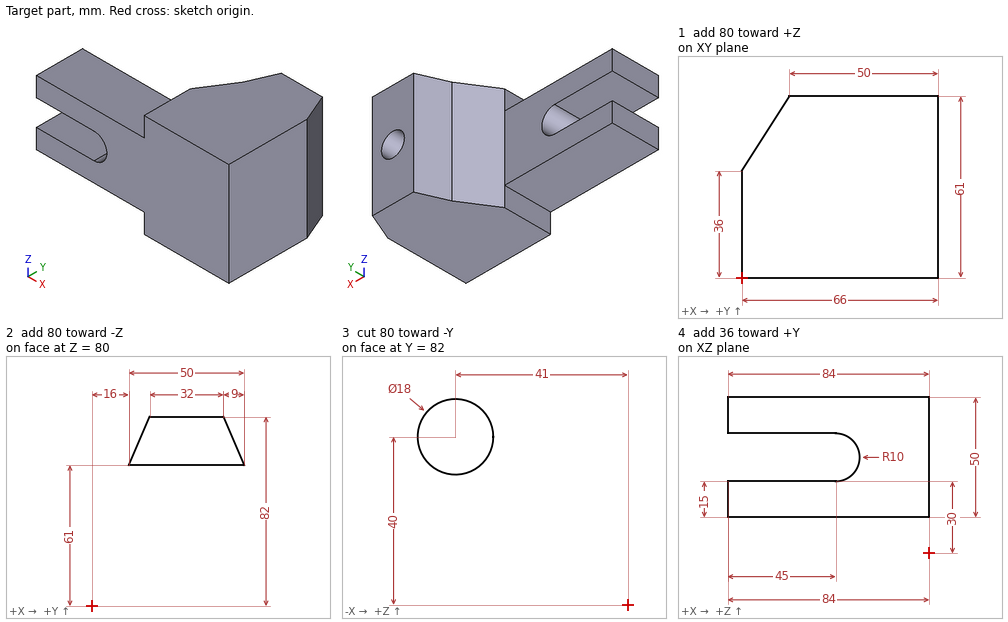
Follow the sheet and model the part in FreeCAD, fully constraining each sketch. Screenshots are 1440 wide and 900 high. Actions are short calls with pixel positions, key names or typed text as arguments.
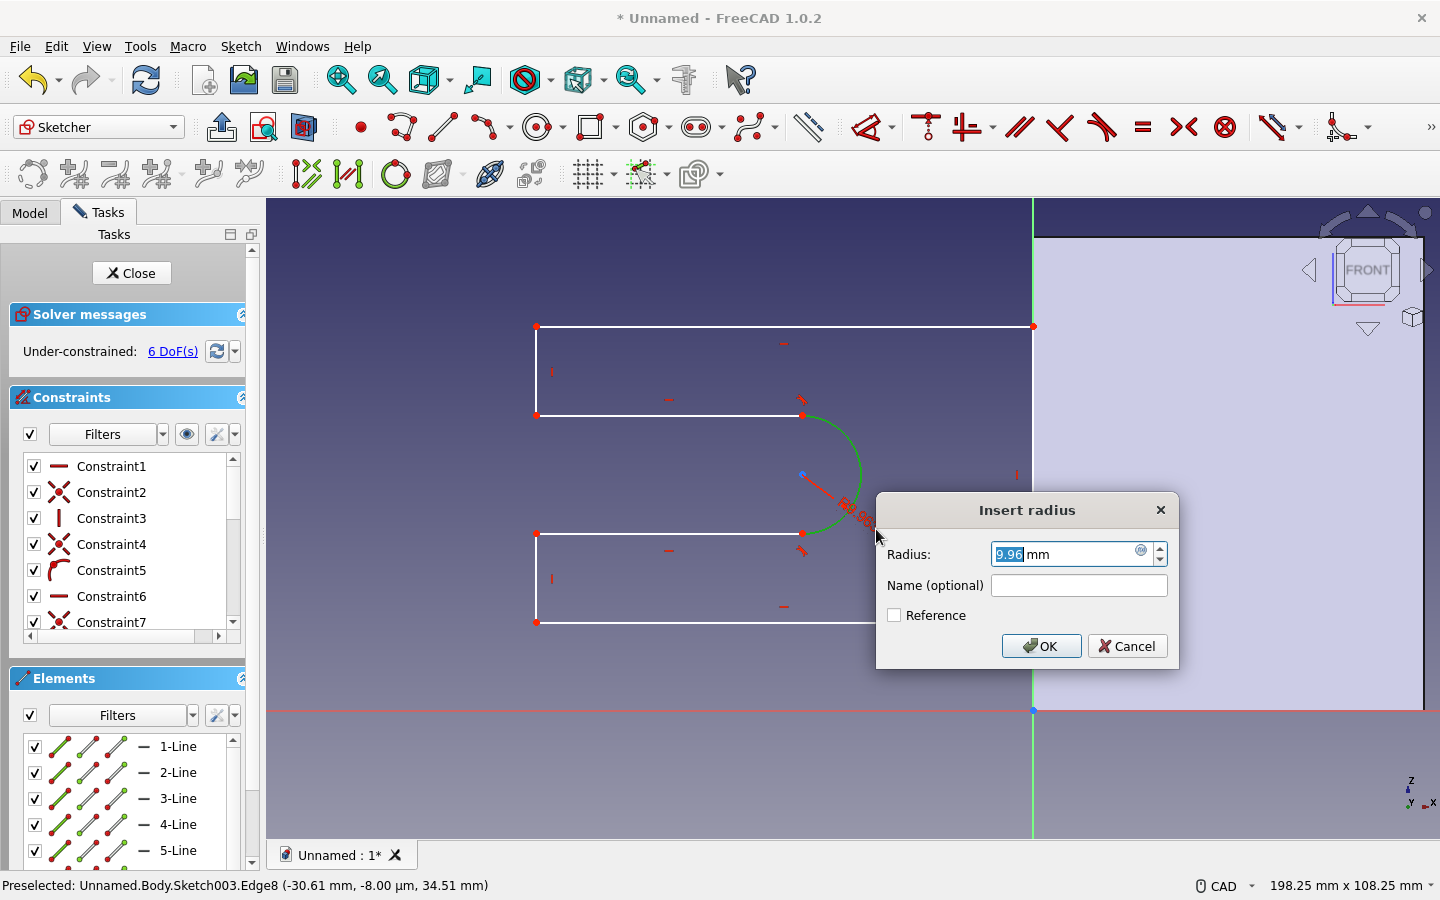
text(10)
key(Return)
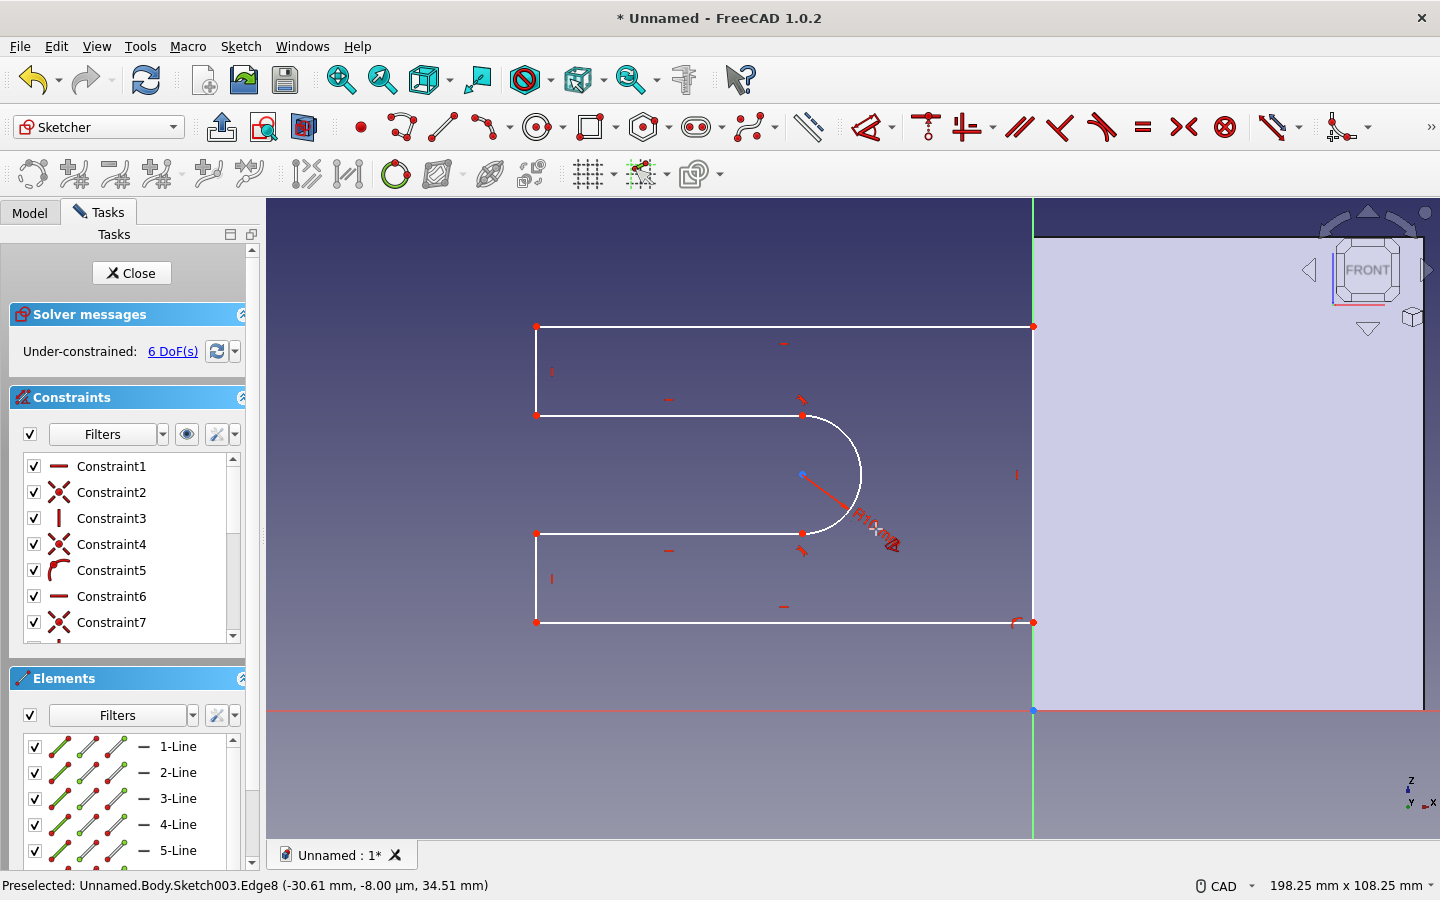
click(722, 534)
click(669, 568)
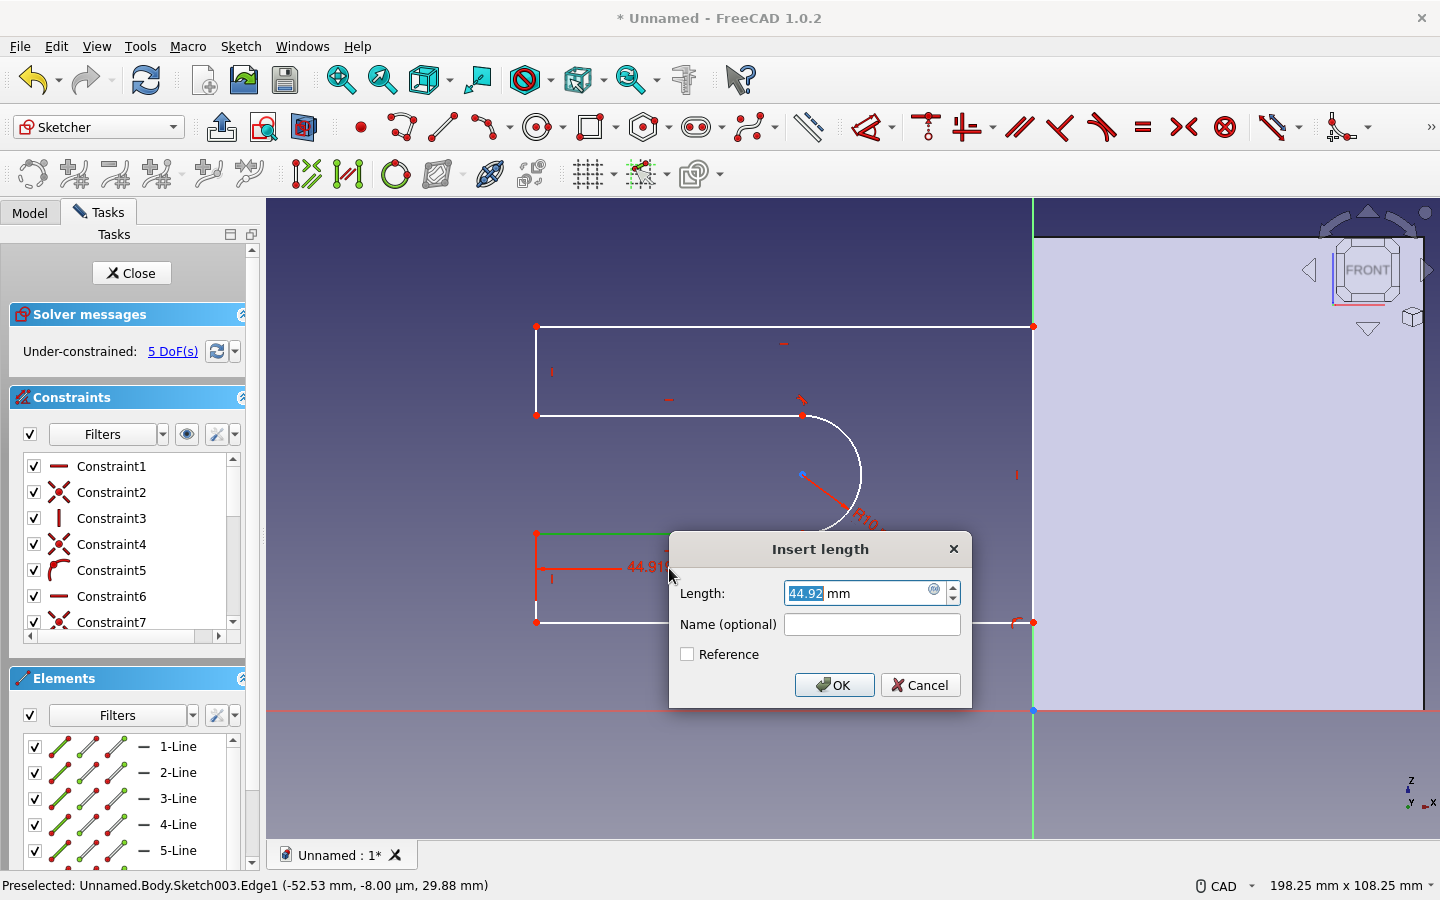
text(45)
key(Return)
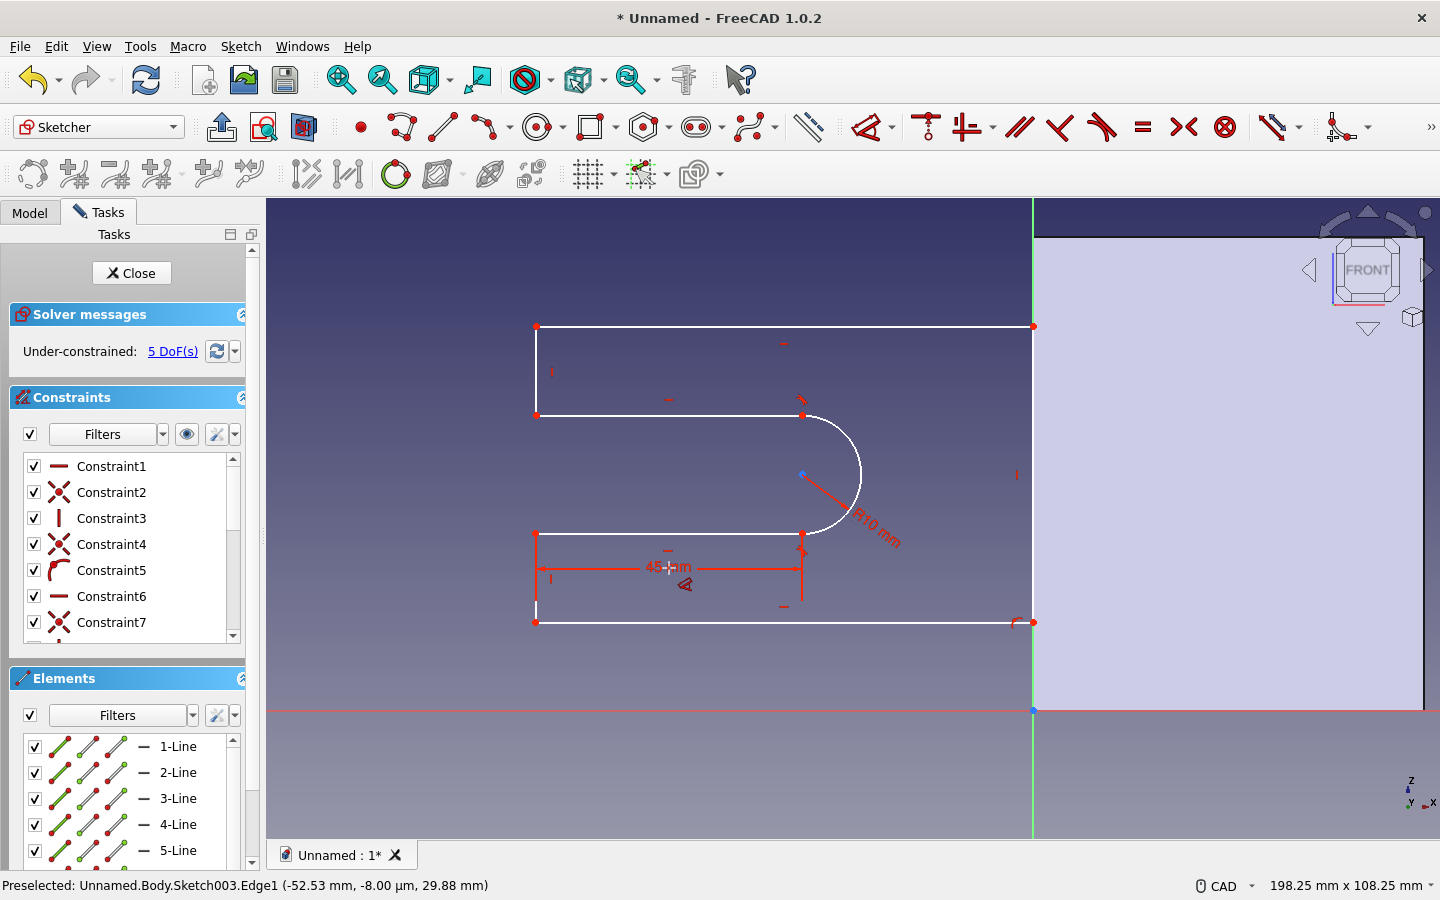
click(536, 561)
click(502, 579)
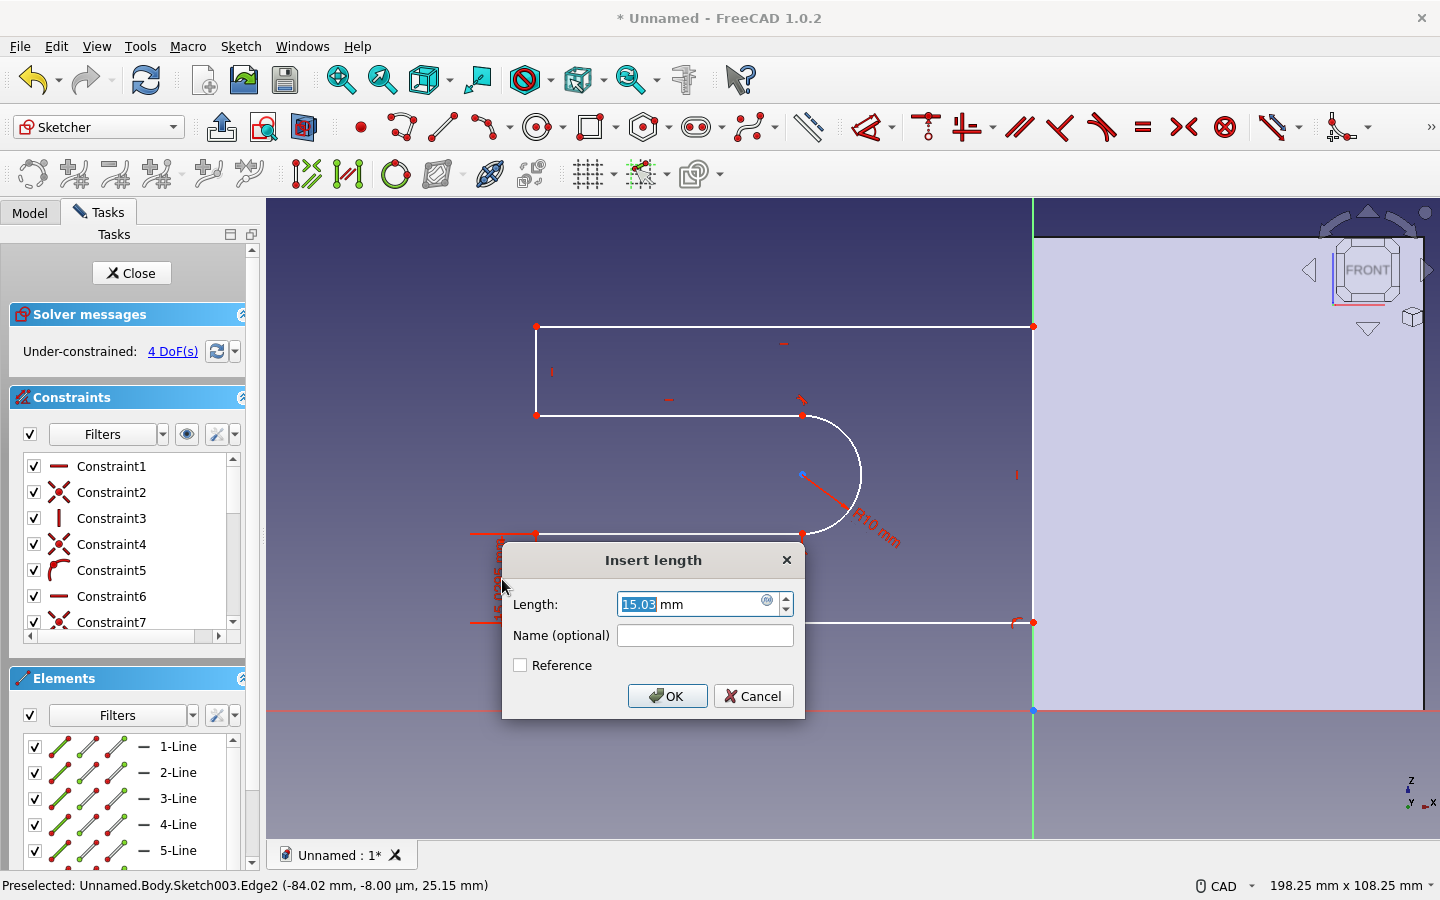
text(15)
key(Return)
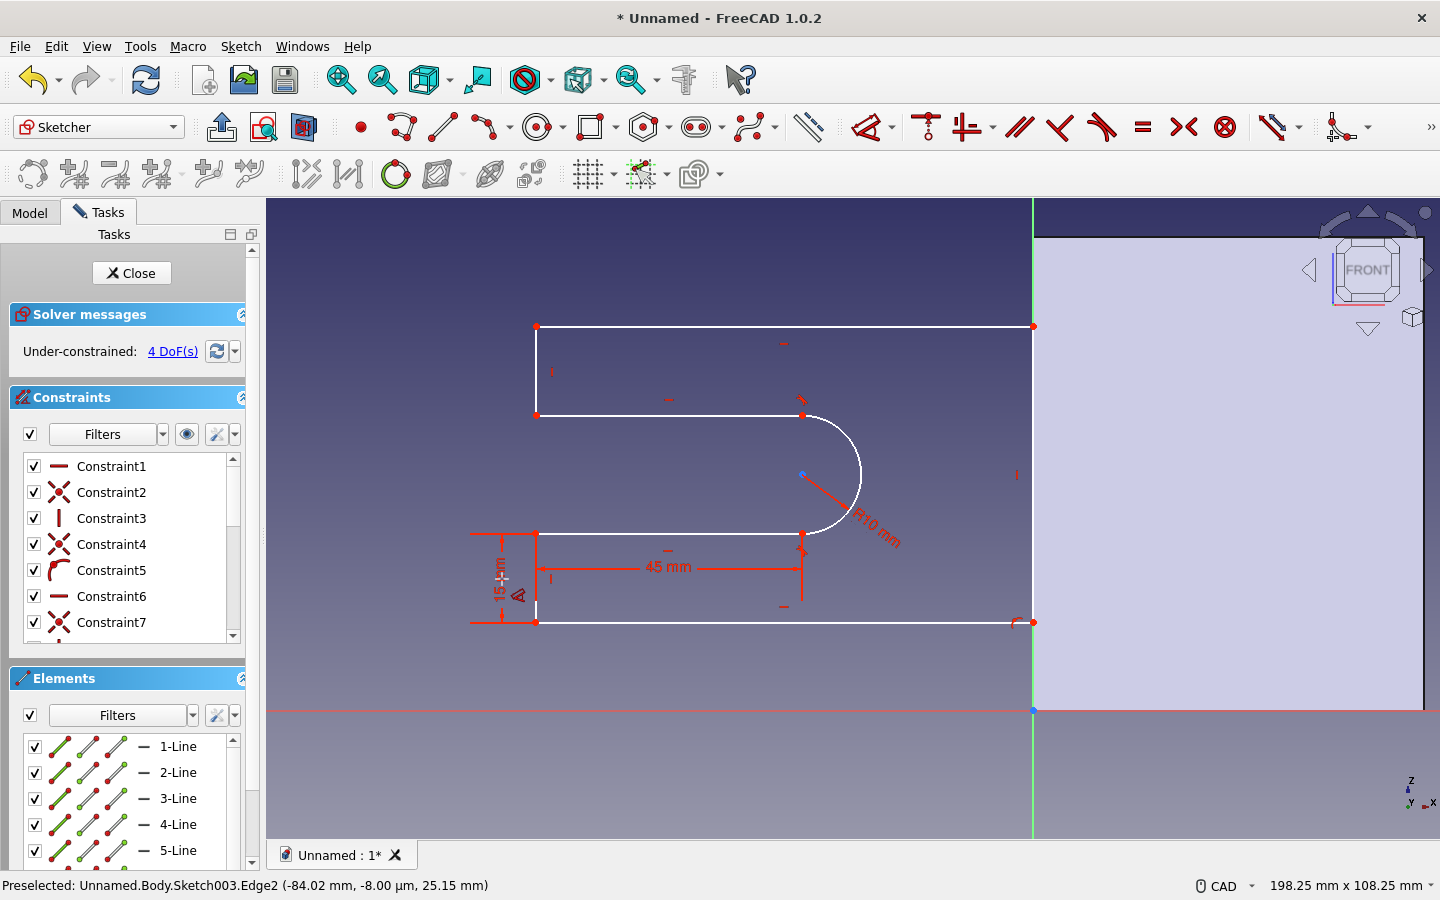
click(685, 623)
click(784, 657)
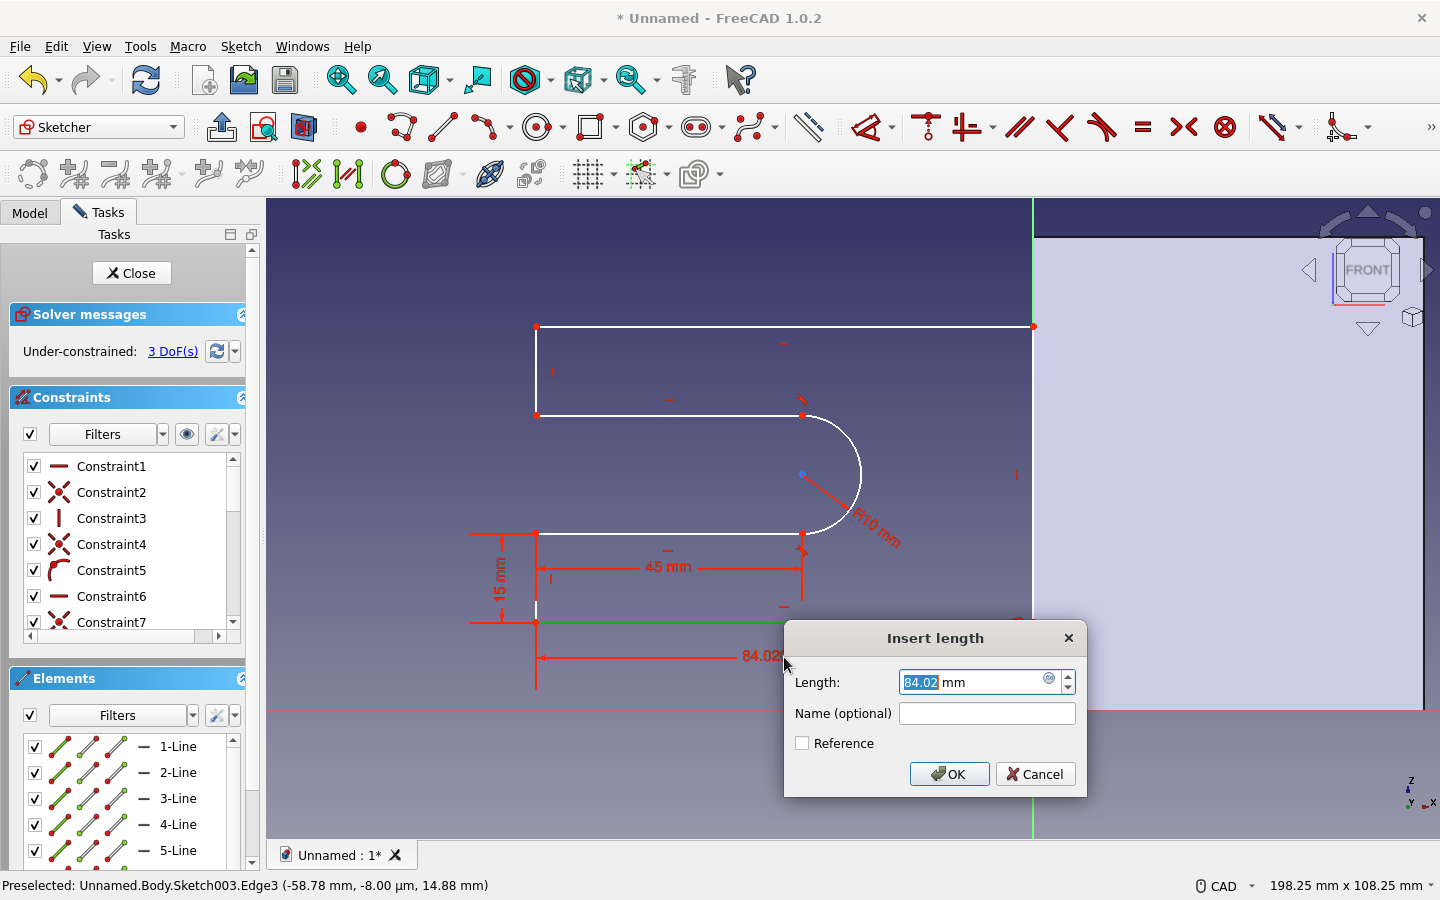
text(84)
key(Return)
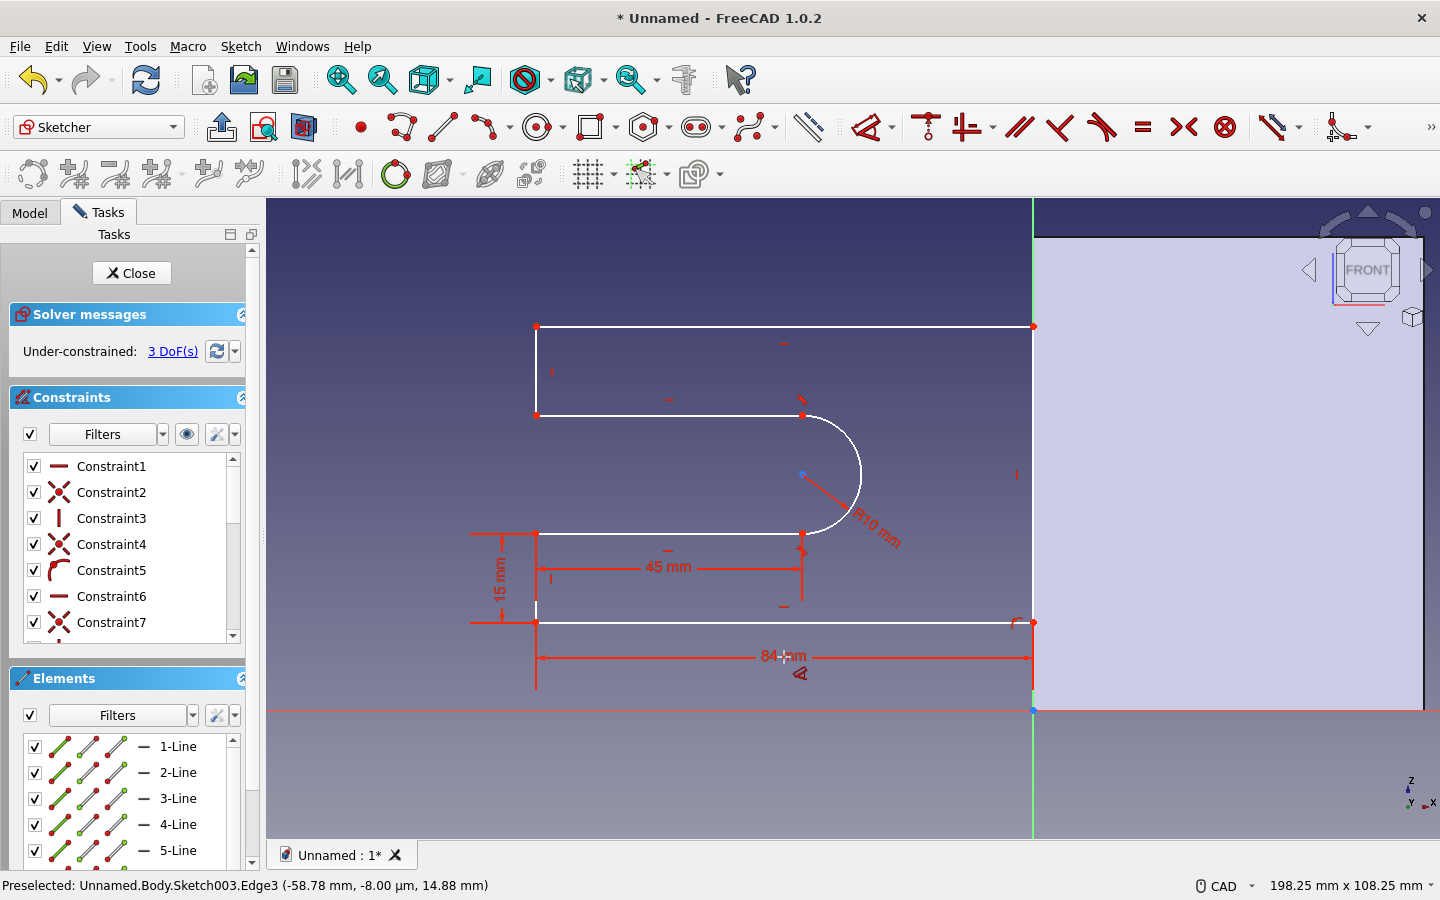
click(1033, 534)
click(1067, 475)